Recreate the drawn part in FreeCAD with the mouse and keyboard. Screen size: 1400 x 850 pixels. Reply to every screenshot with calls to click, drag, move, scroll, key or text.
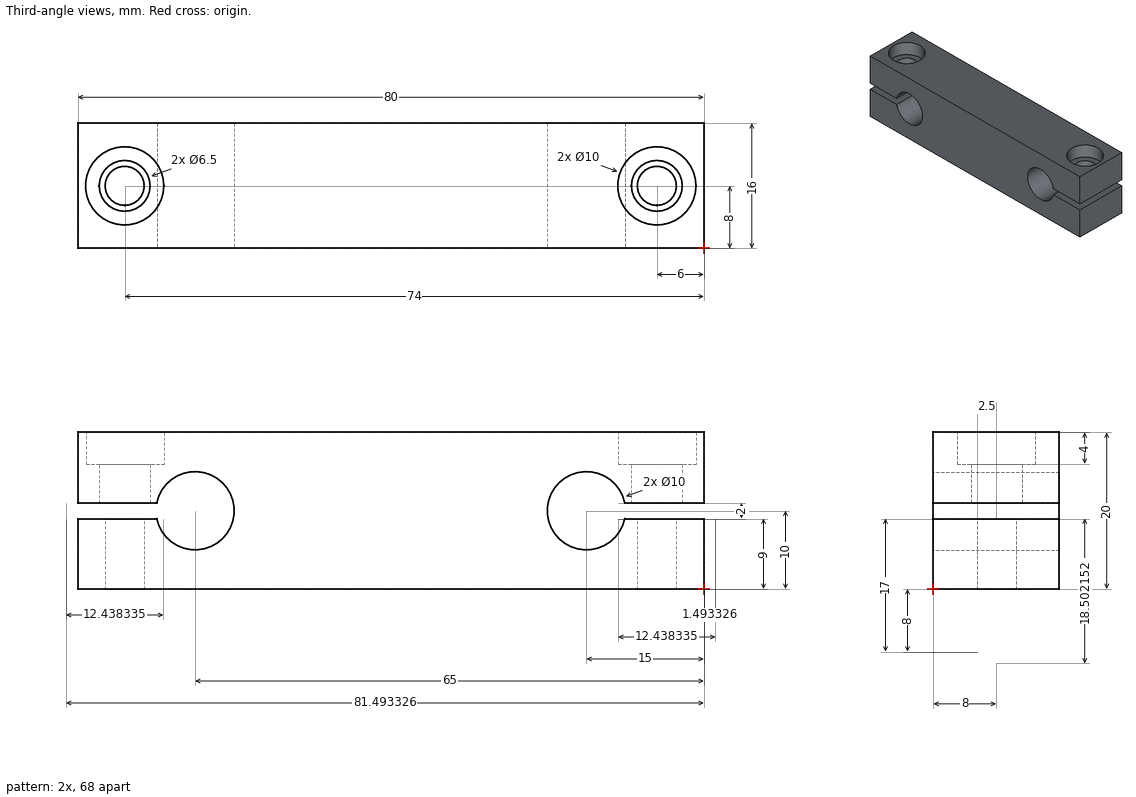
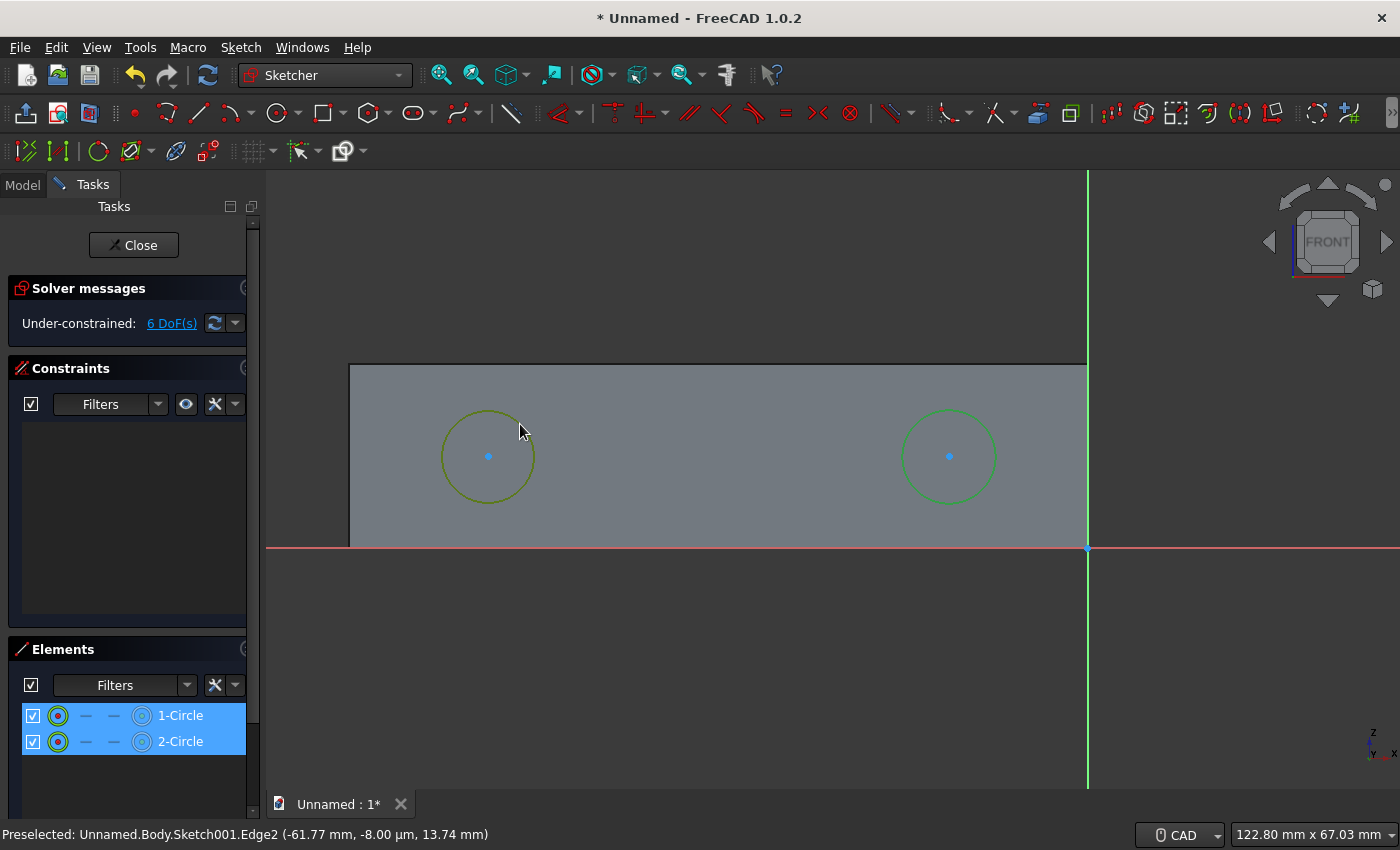
click(786, 114)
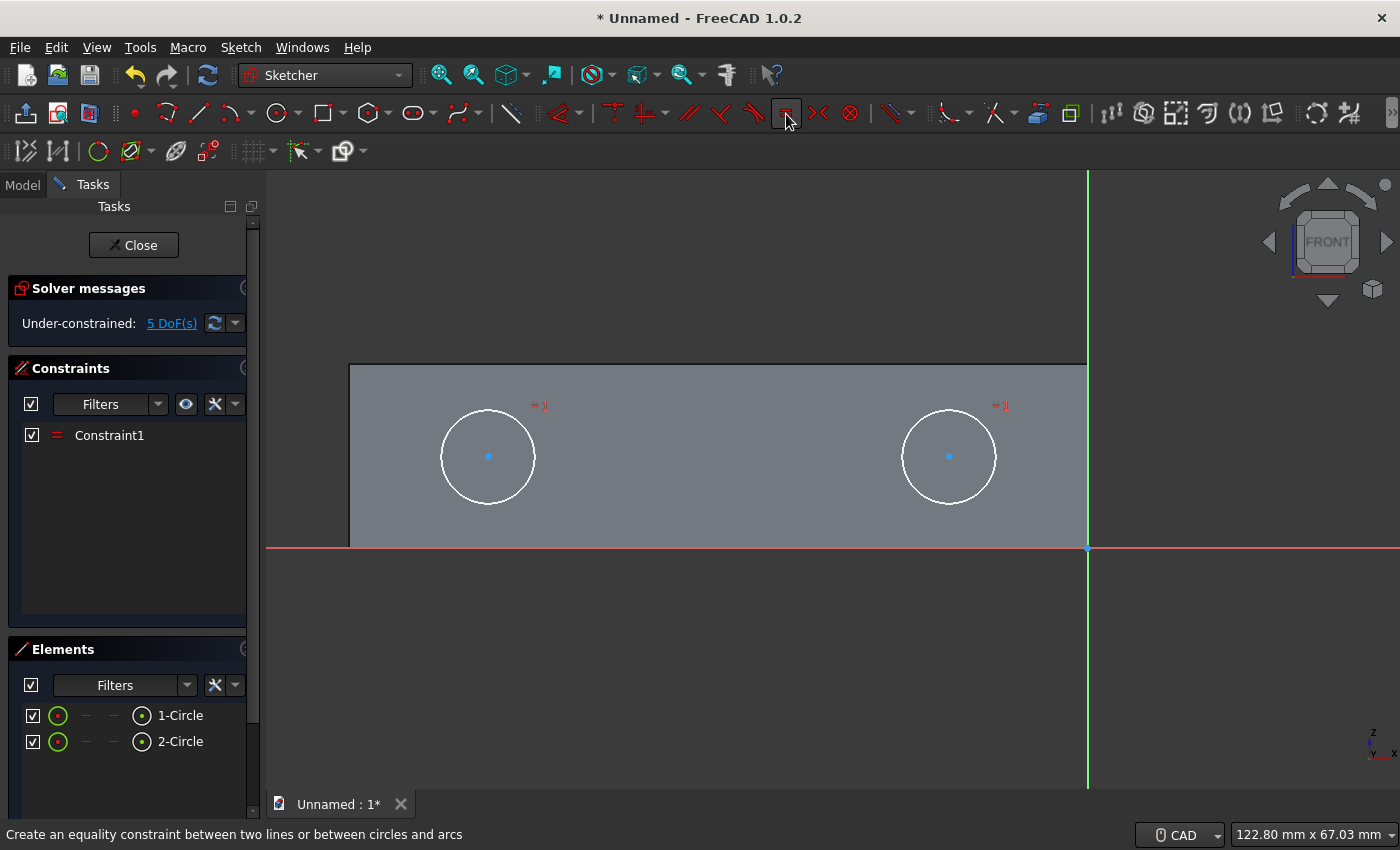
click(558, 114)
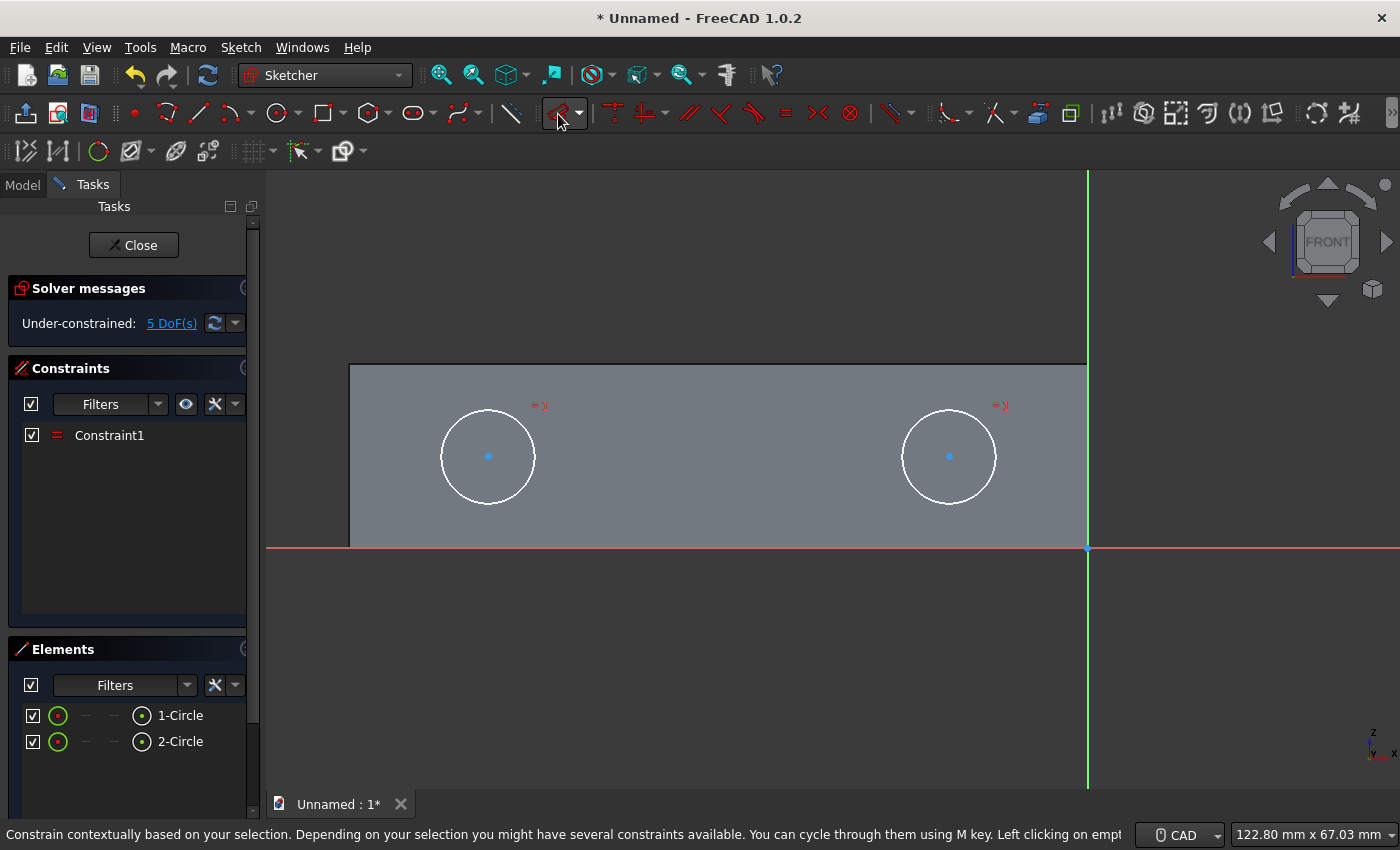
click(982, 424)
click(1005, 401)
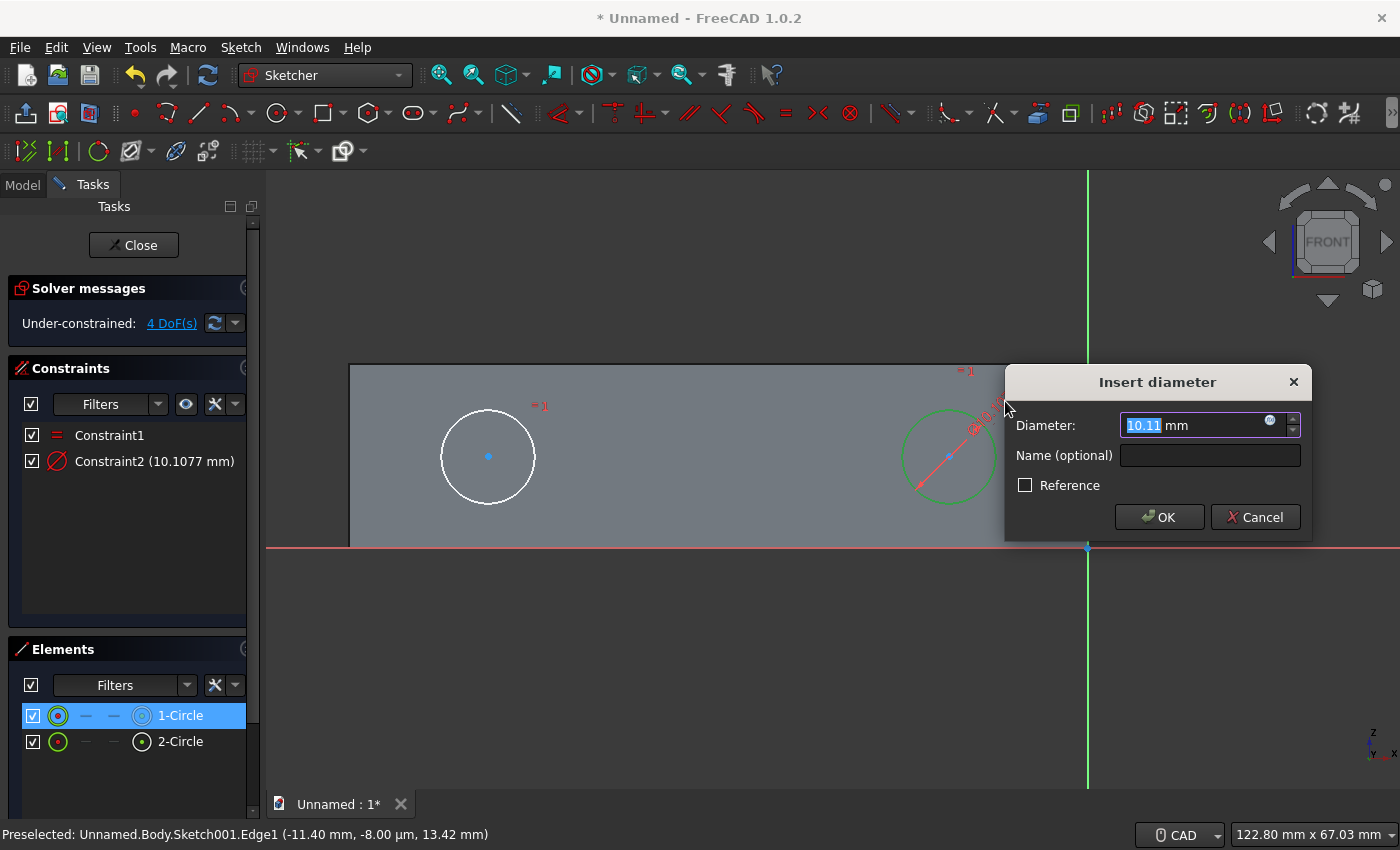
text(10)
key(Return)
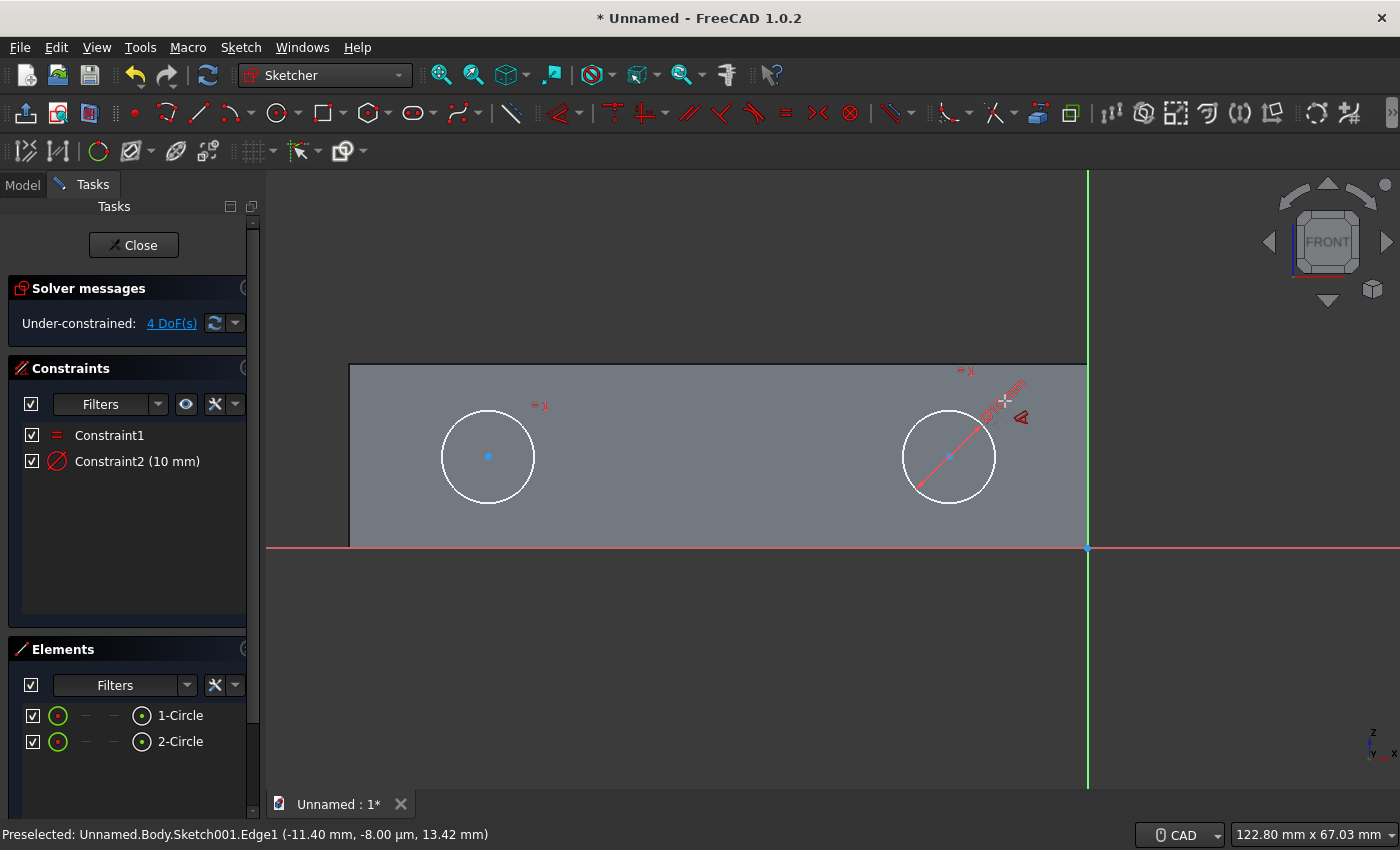
click(949, 457)
click(1018, 582)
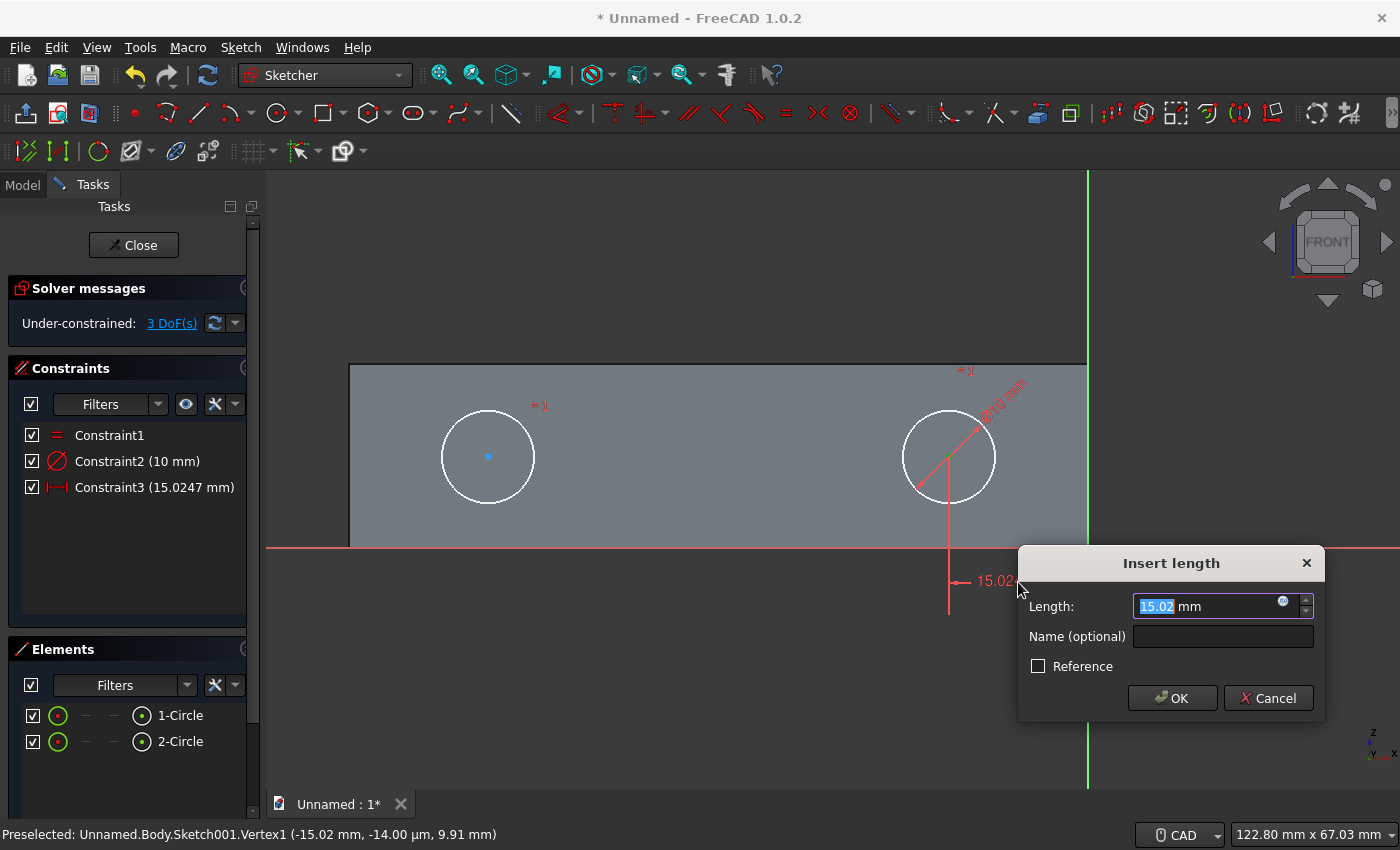
text(15)
key(Return)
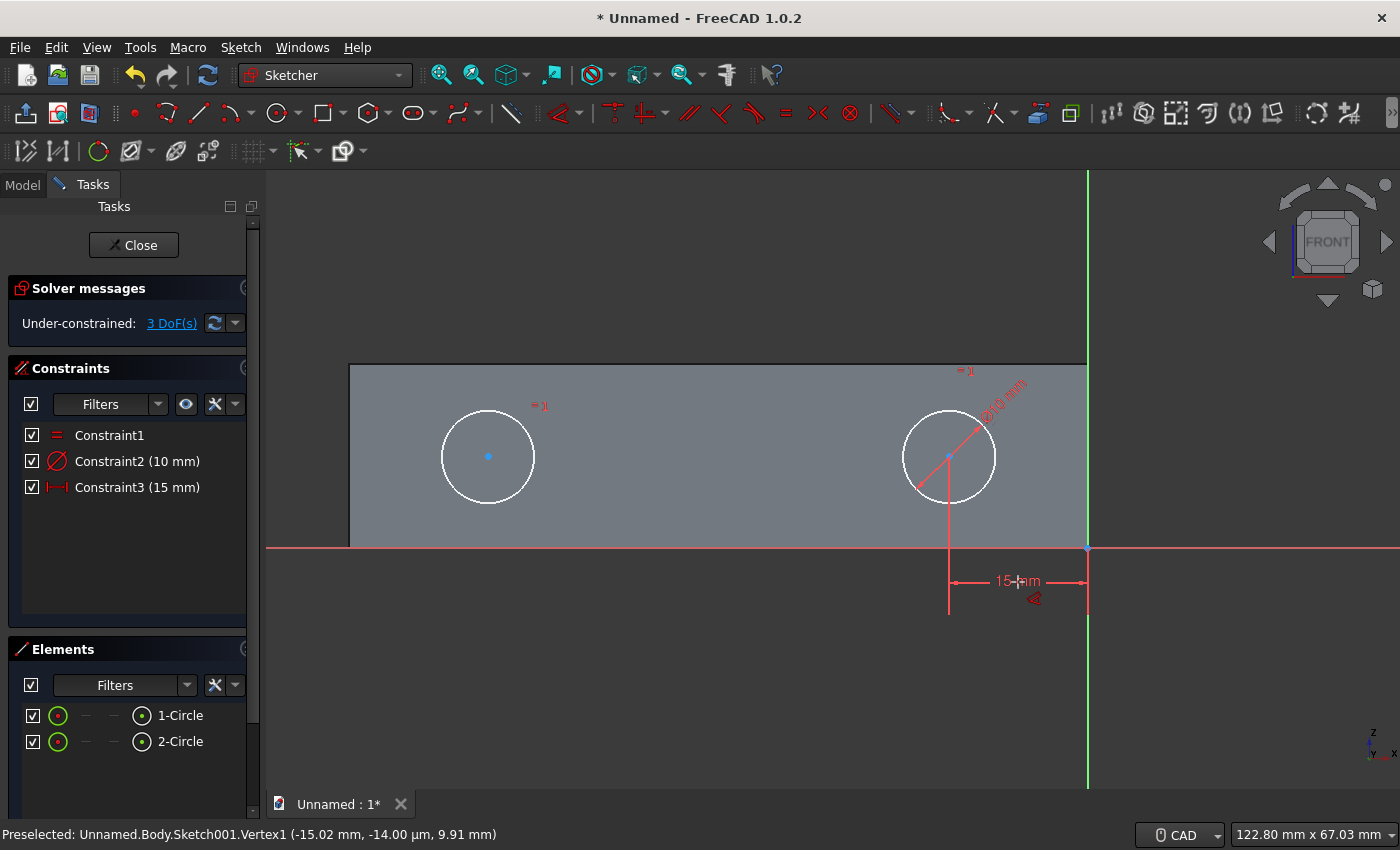
click(949, 457)
click(1122, 503)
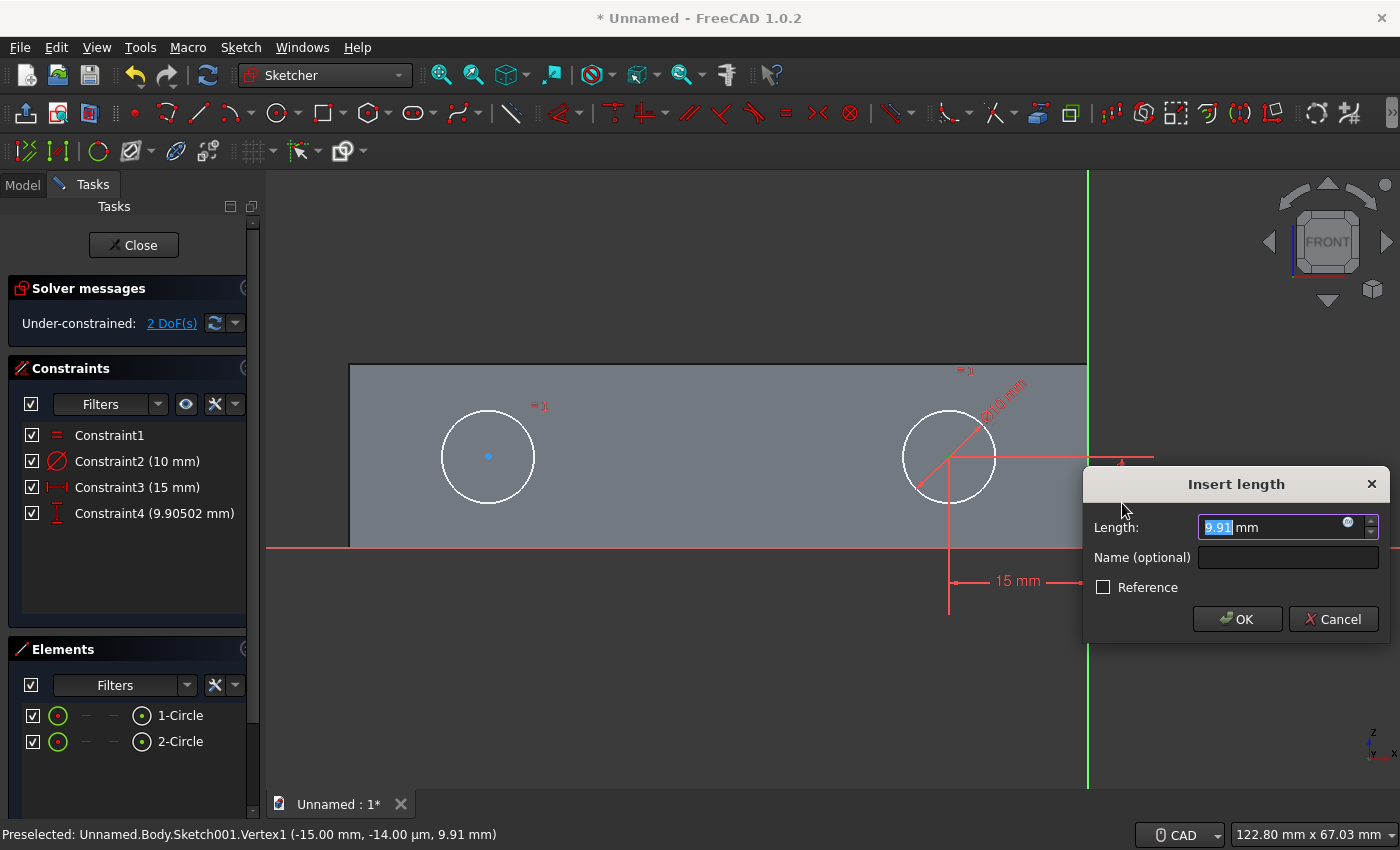
text(10)
key(Return)